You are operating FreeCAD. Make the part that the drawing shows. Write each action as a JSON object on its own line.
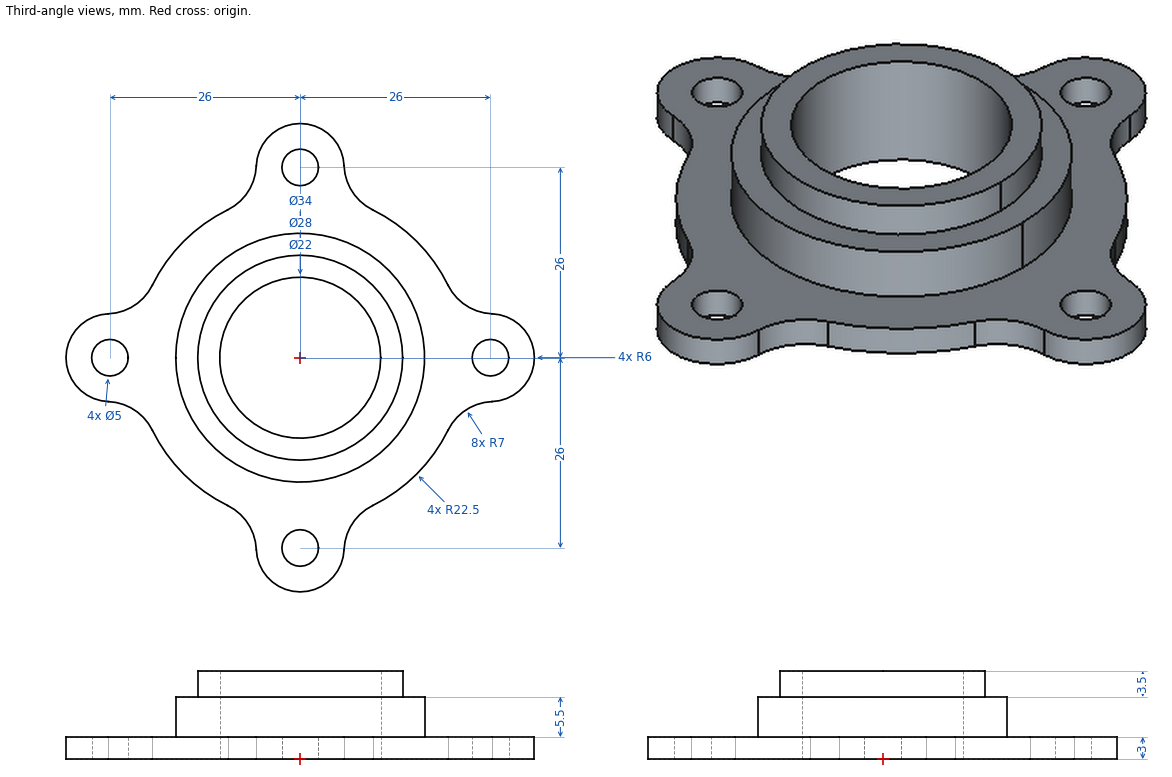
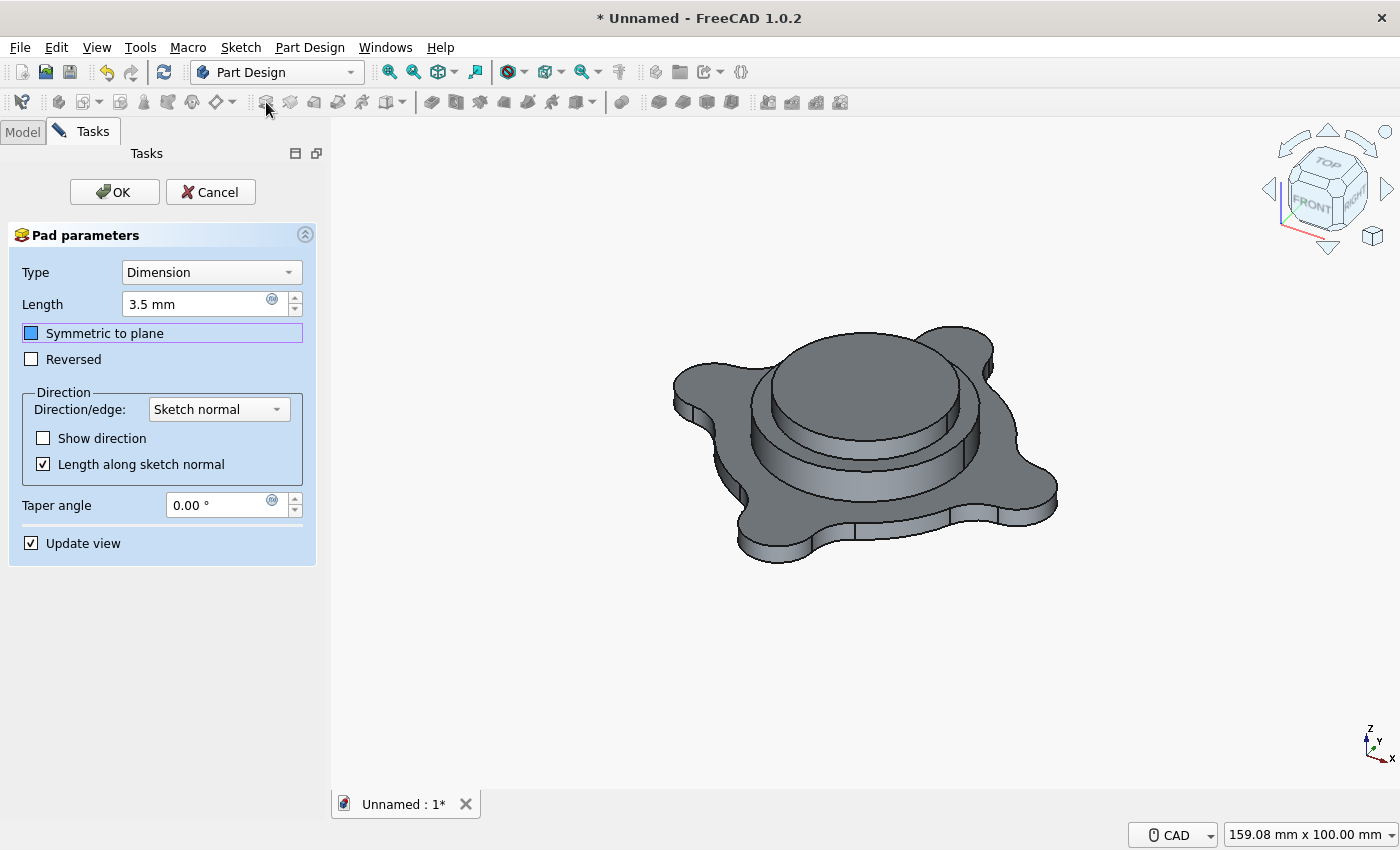
{"action": "left_click", "coordinate": [115, 192]}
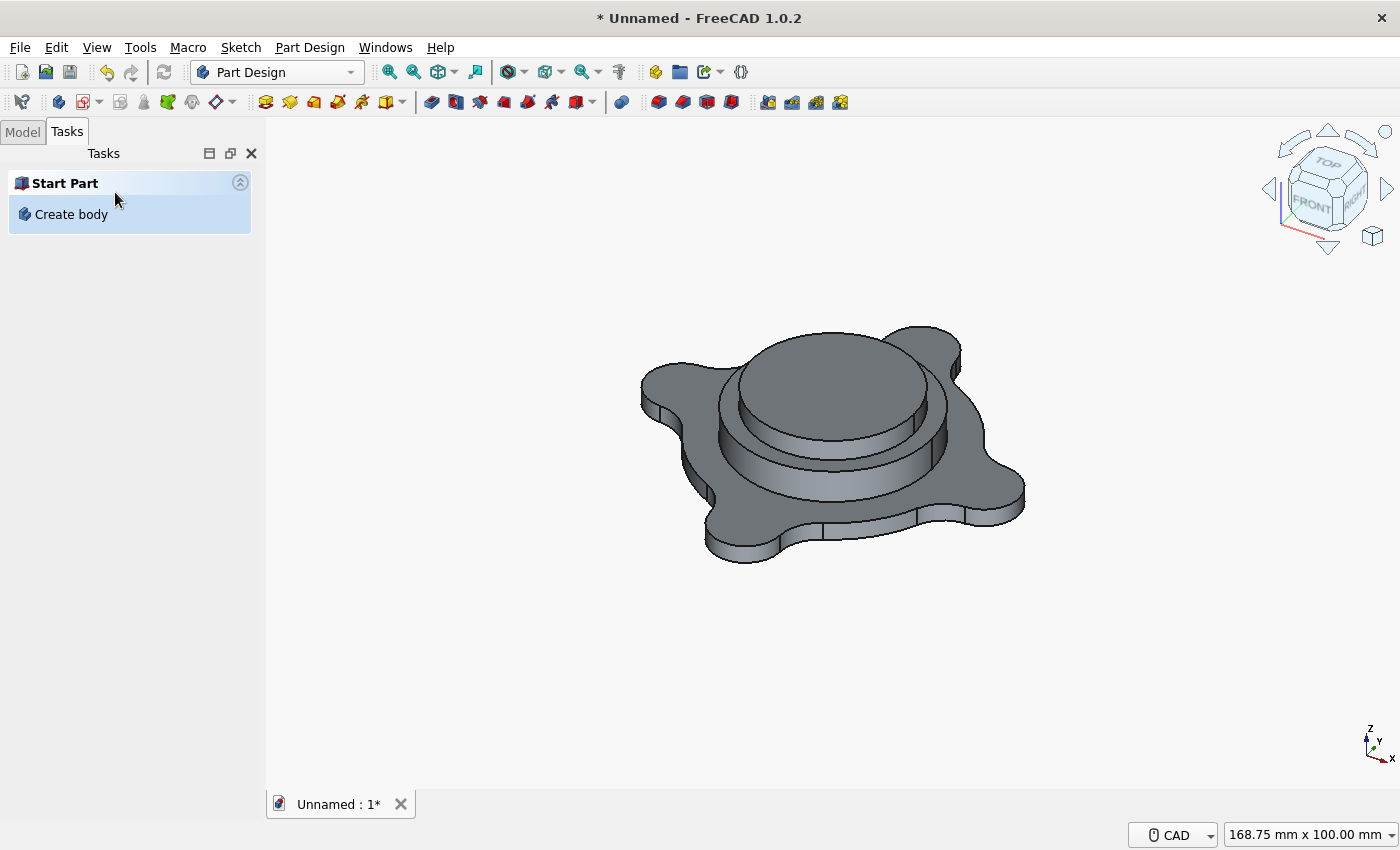
{"action": "left_click", "coordinate": [833, 386]}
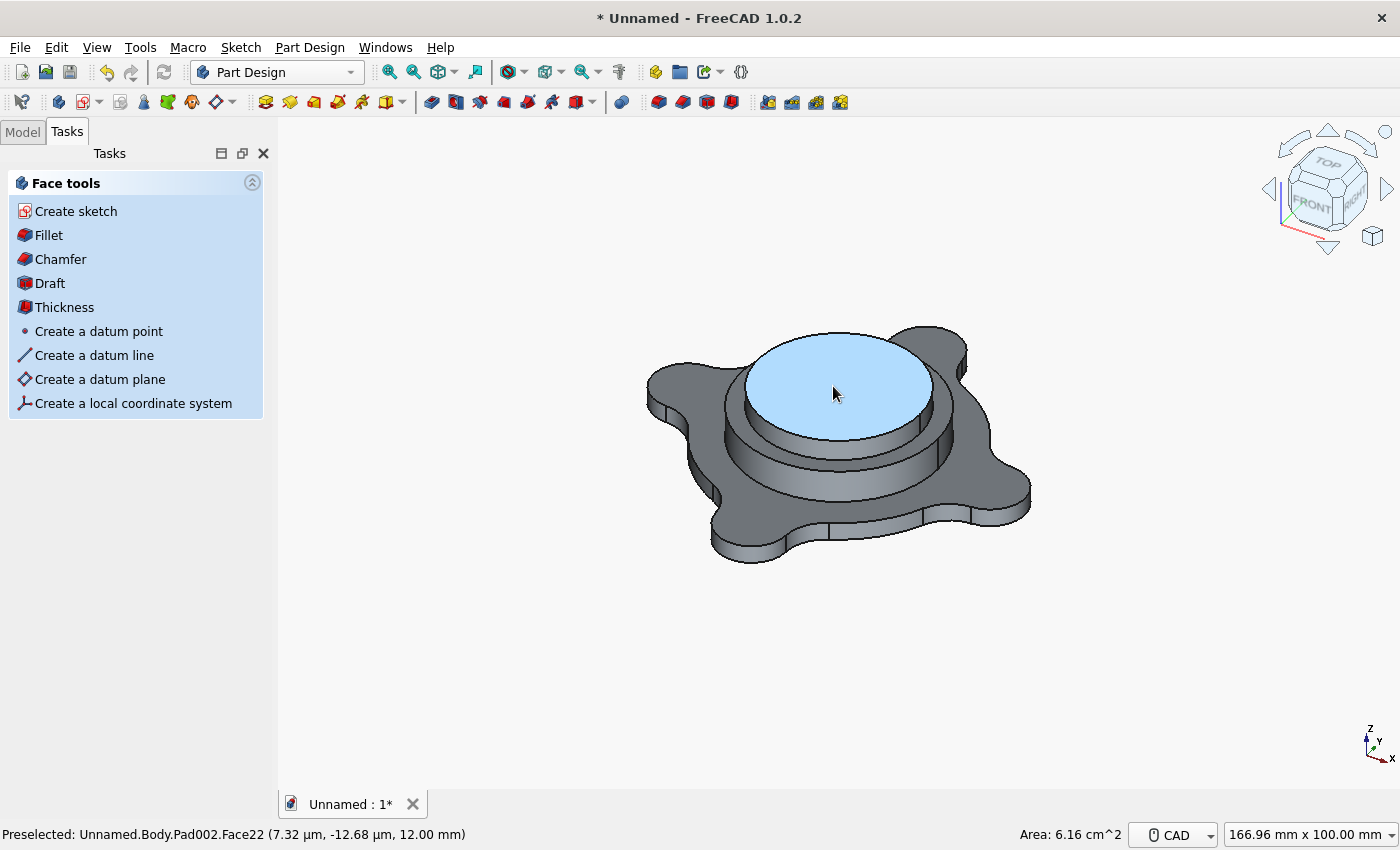
{"action": "left_click", "coordinate": [84, 102]}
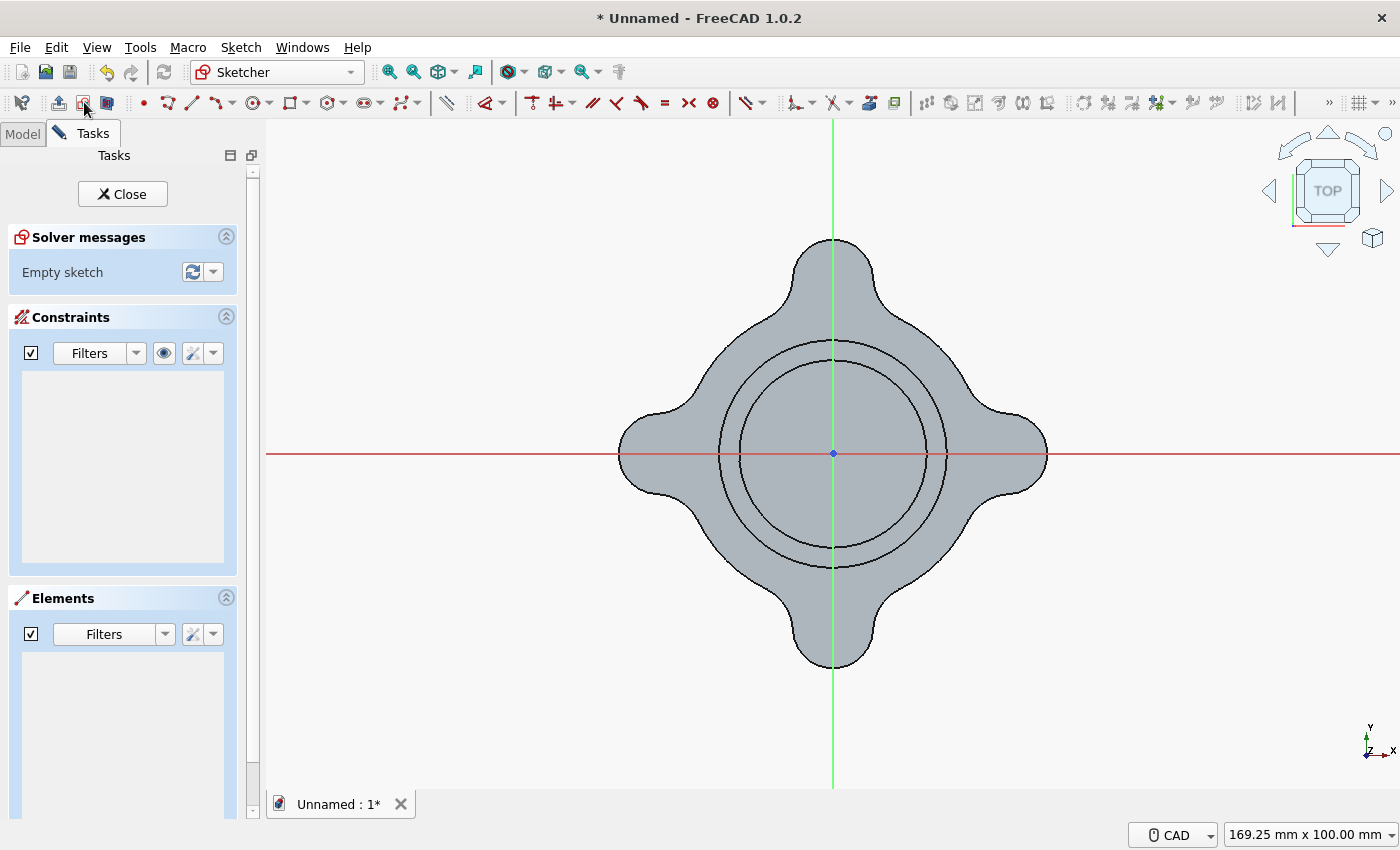
{"action": "scroll", "coordinate": [873, 454], "scroll_direction": "up", "scroll_amount": 5}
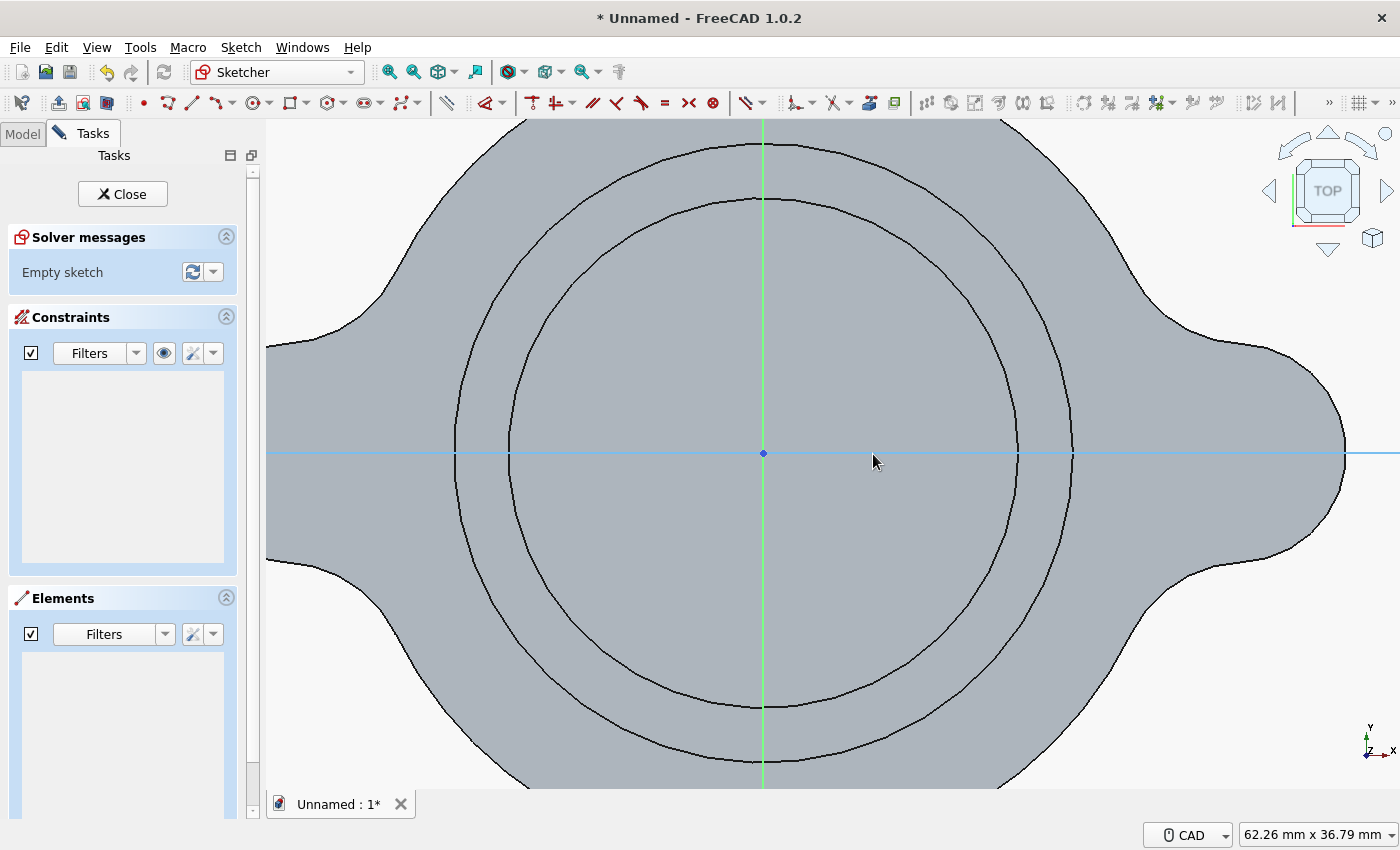
{"action": "left_click", "coordinate": [254, 104]}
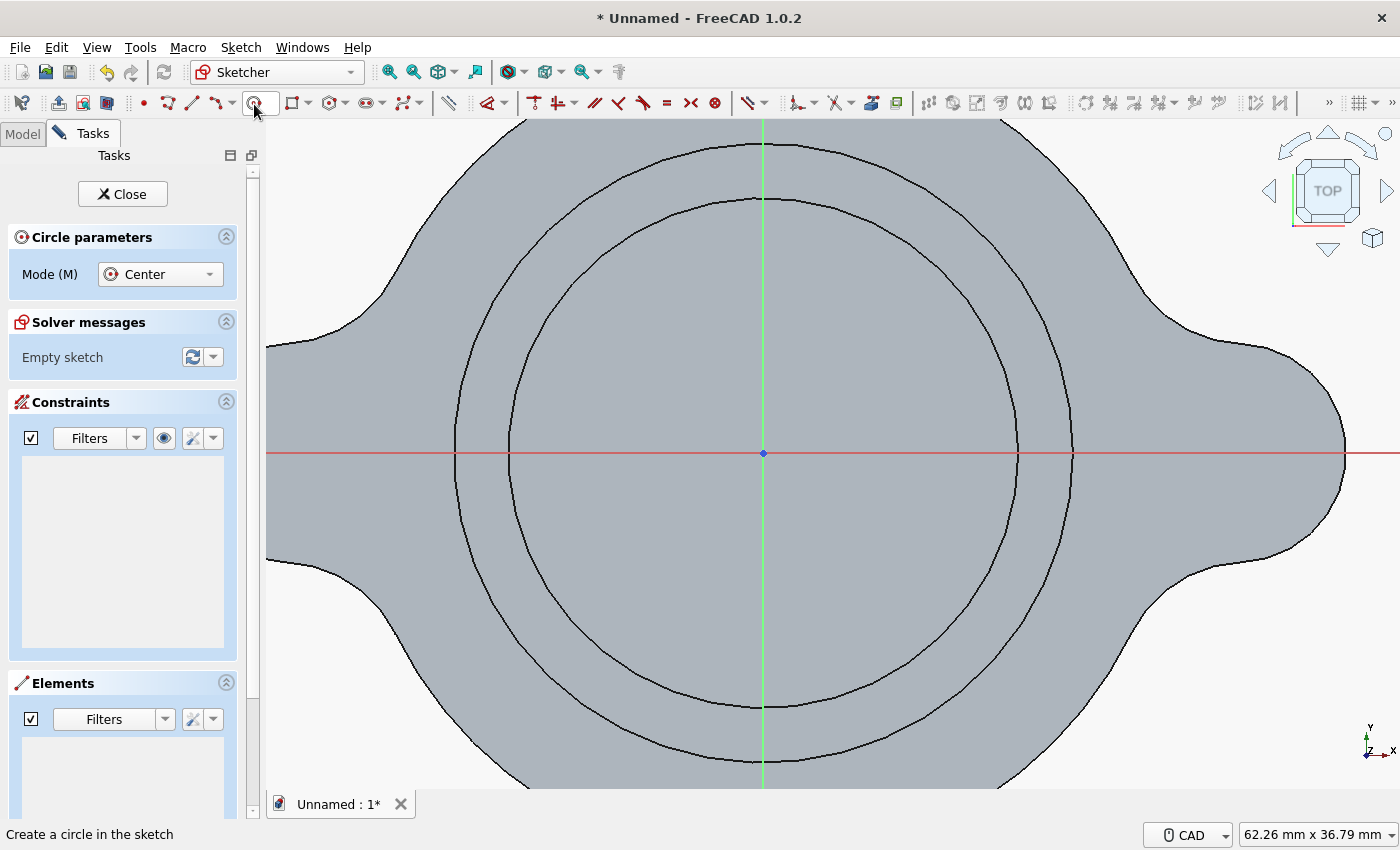
{"action": "left_click", "coordinate": [763, 453]}
{"action": "mouse_move", "coordinate": [905, 311]}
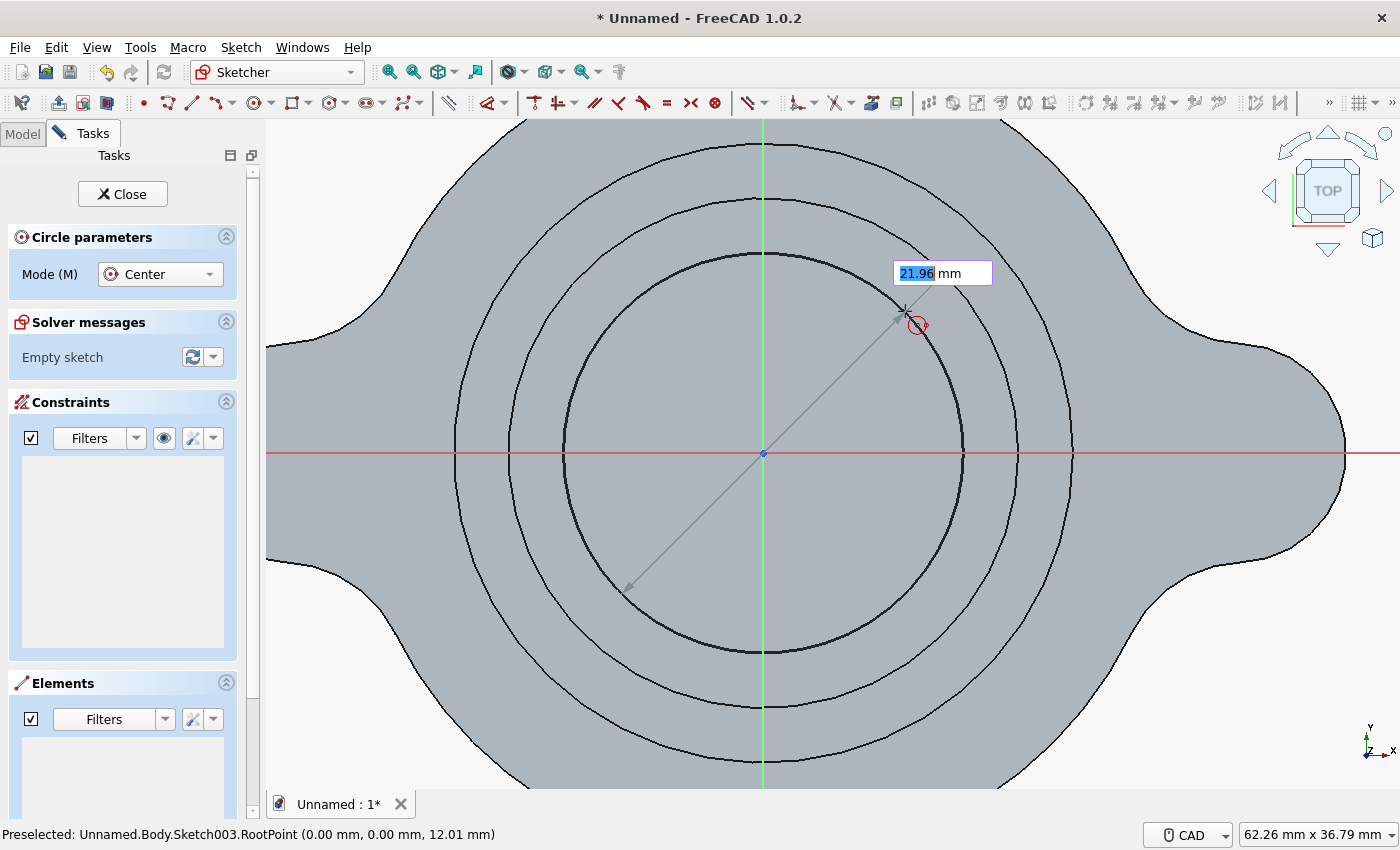
{"action": "type", "text": "22"}
{"action": "key", "text": "Return"}
{"action": "key", "text": "Escape"}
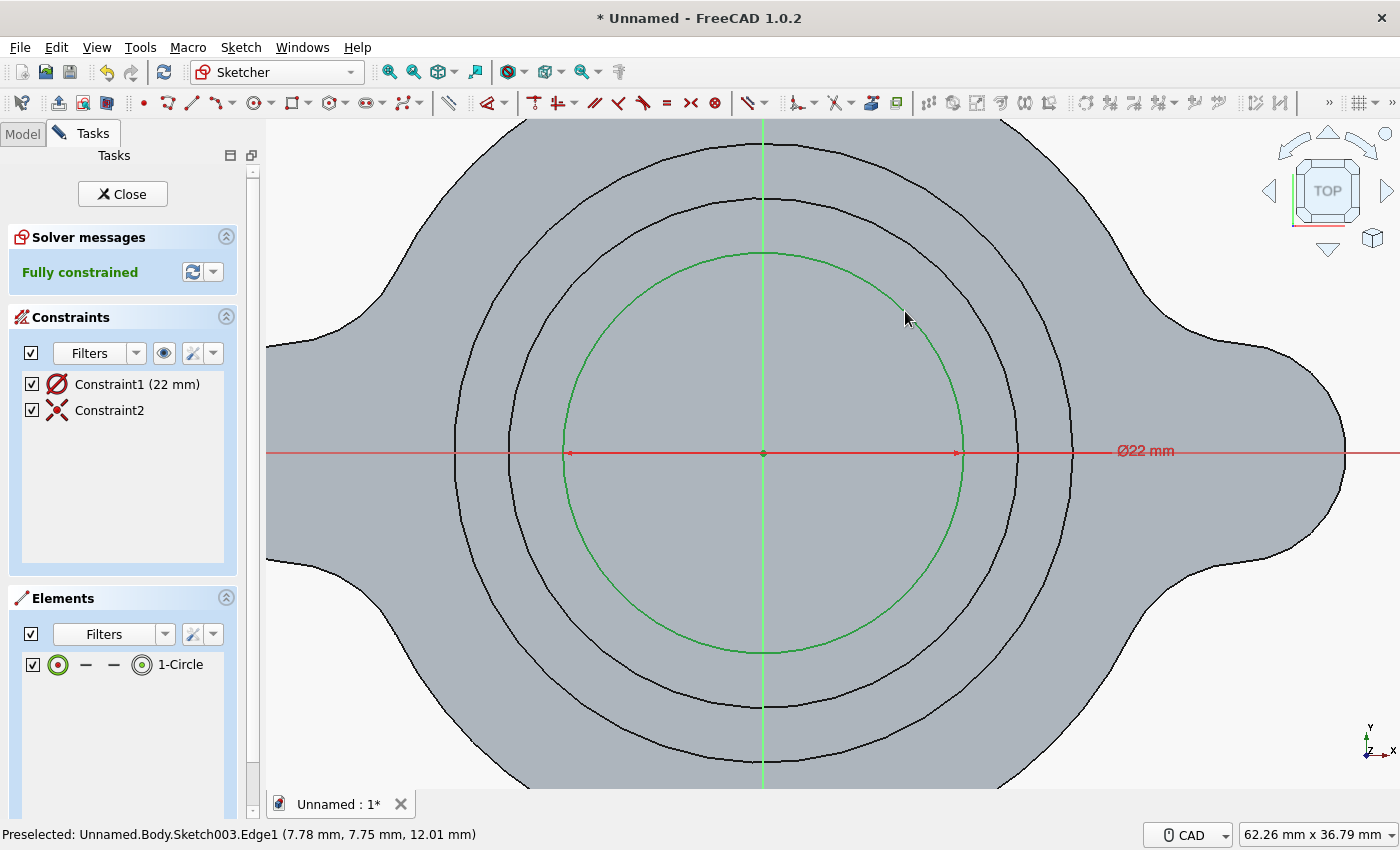
{"action": "left_click", "coordinate": [123, 194]}